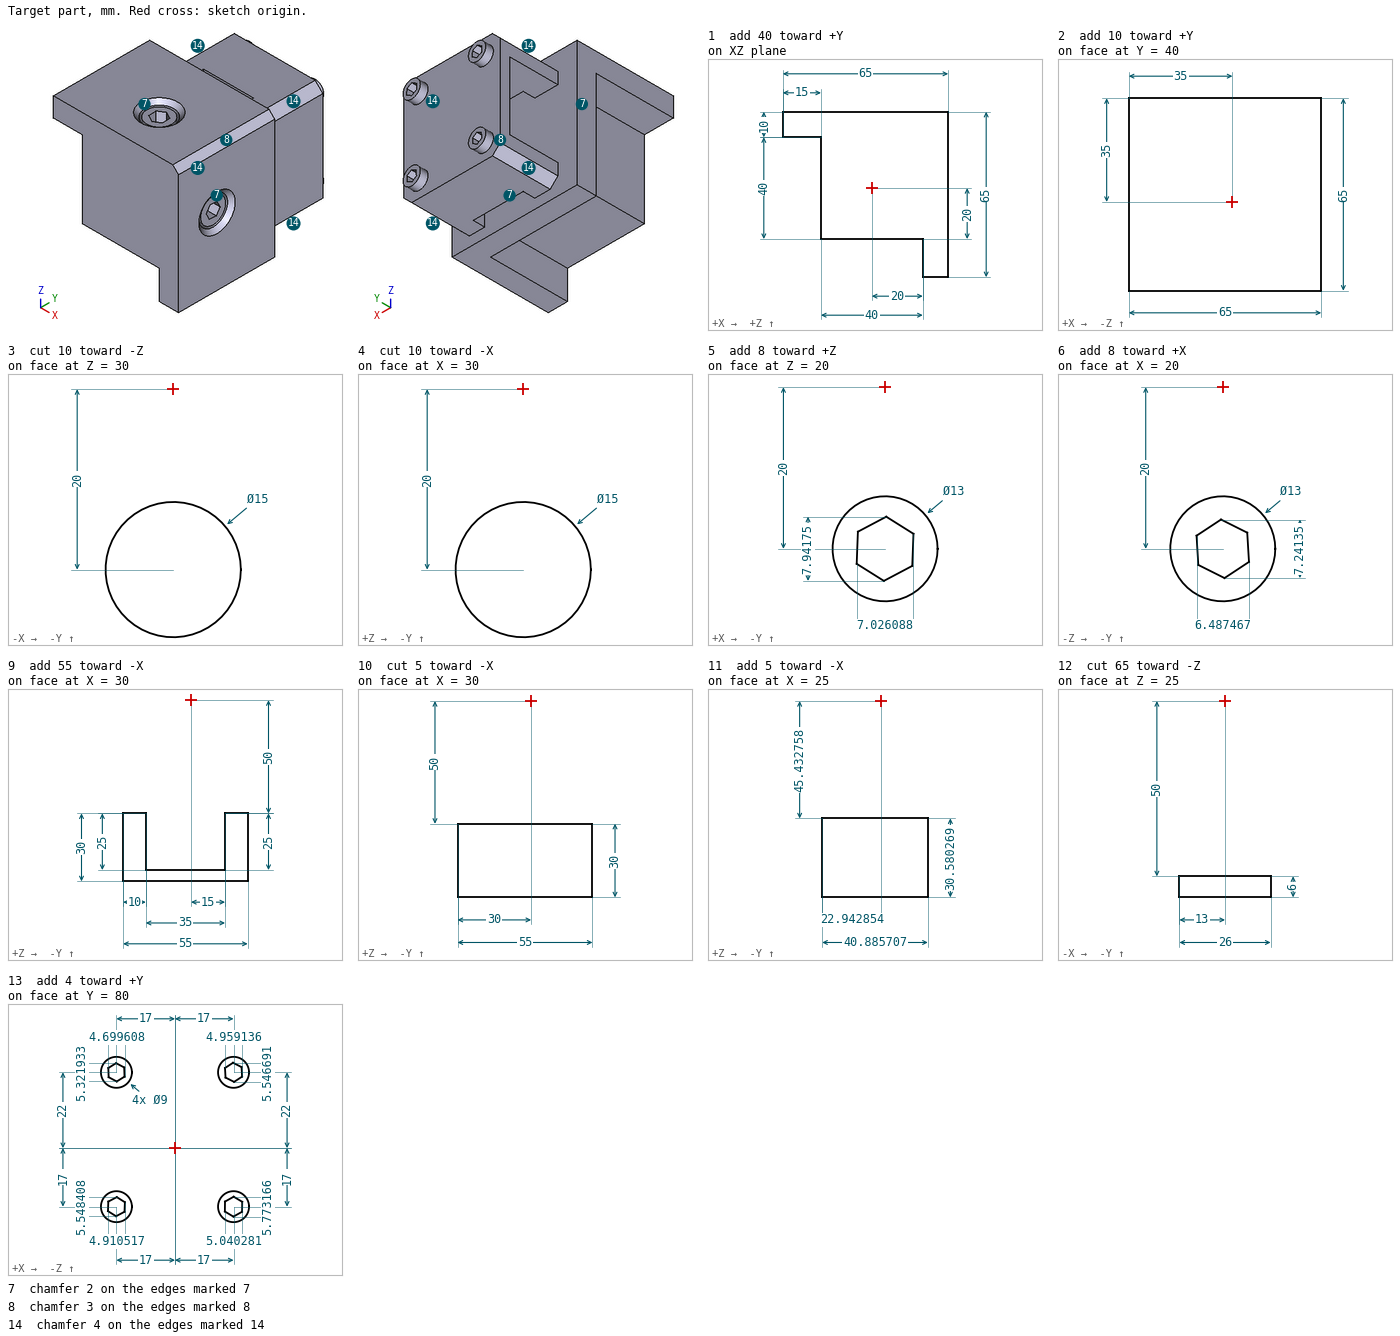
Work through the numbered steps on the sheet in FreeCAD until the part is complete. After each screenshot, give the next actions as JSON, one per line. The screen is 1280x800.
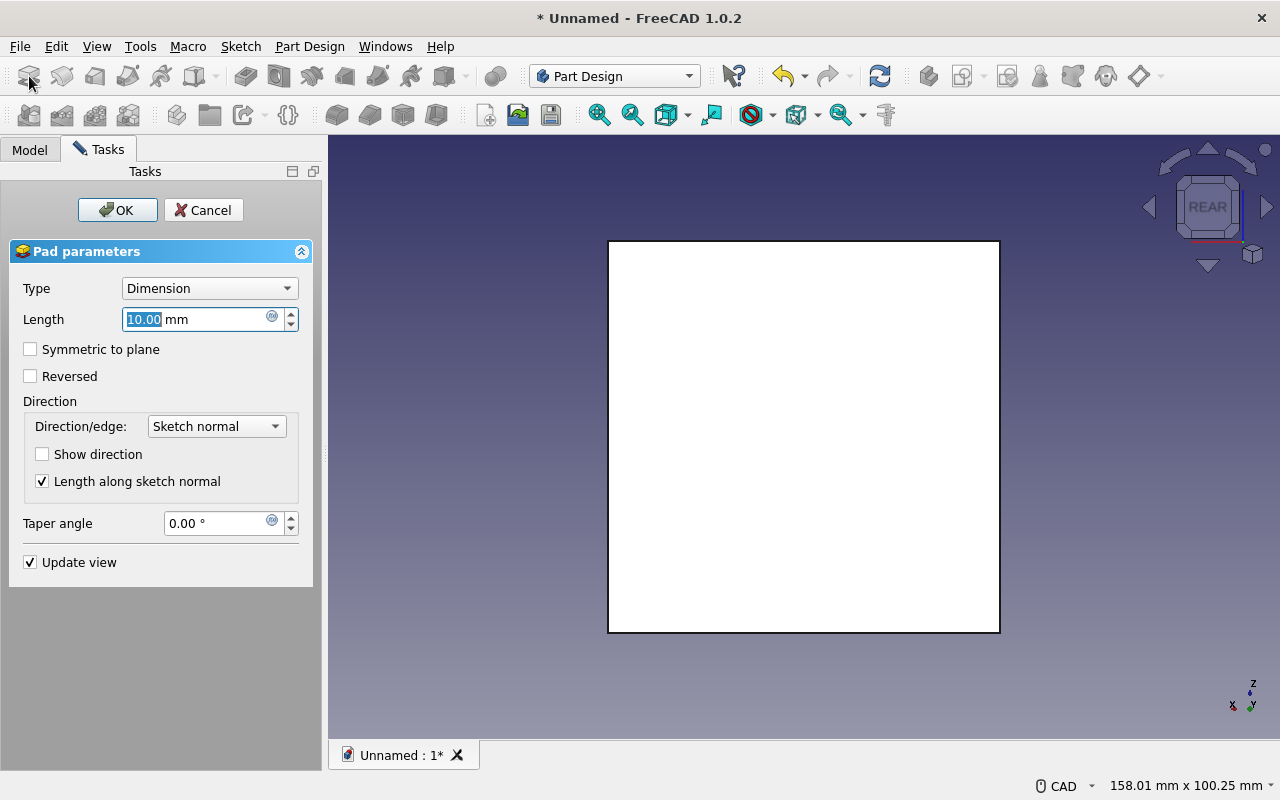
{"action": "type", "text": "10"}
{"action": "key", "text": "Tab"}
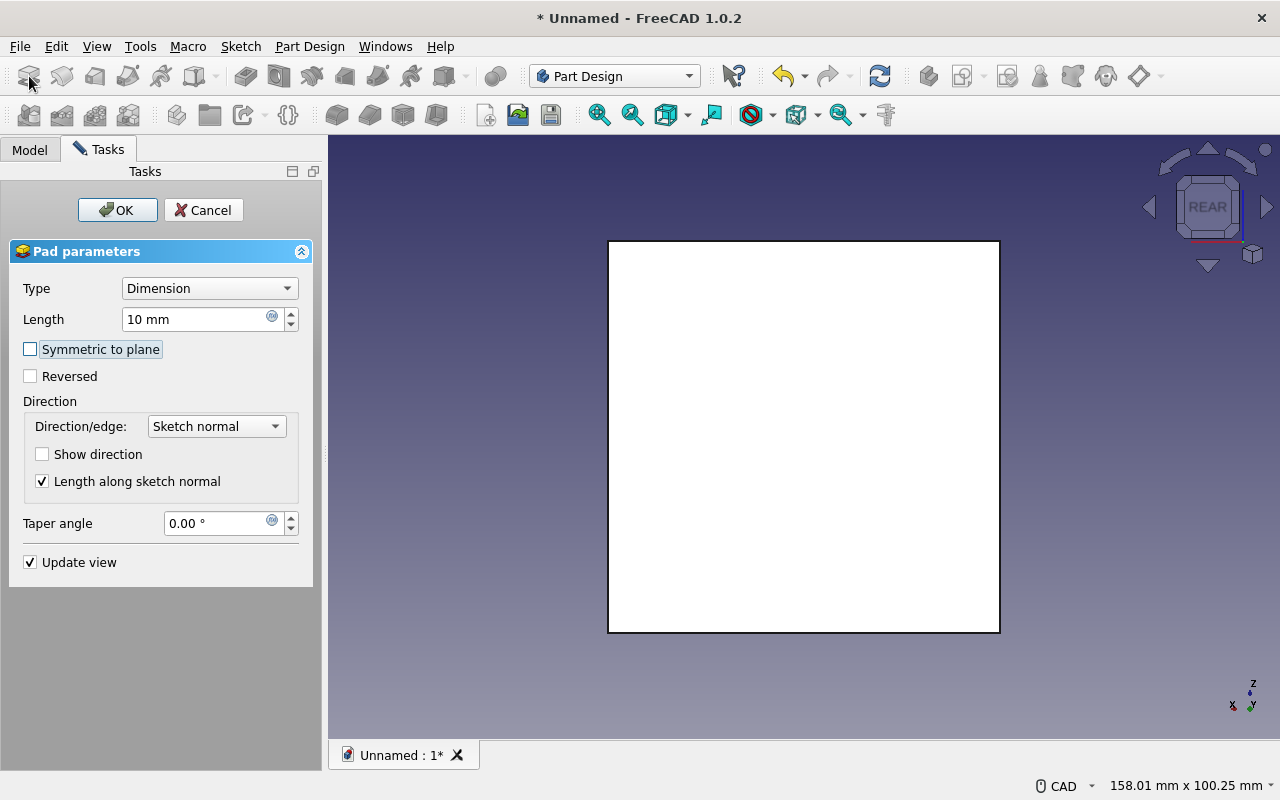
{"action": "left_click", "coordinate": [118, 210]}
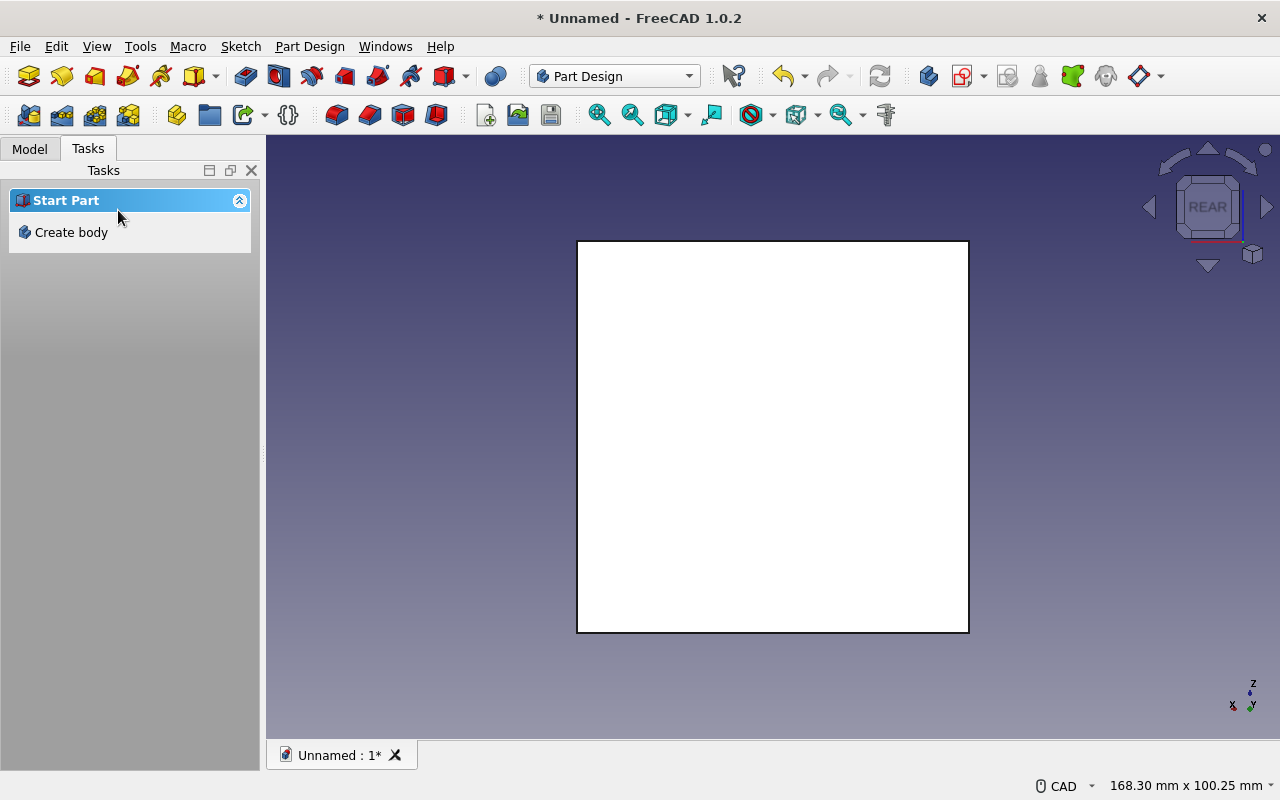
{"action": "key", "text": "0"}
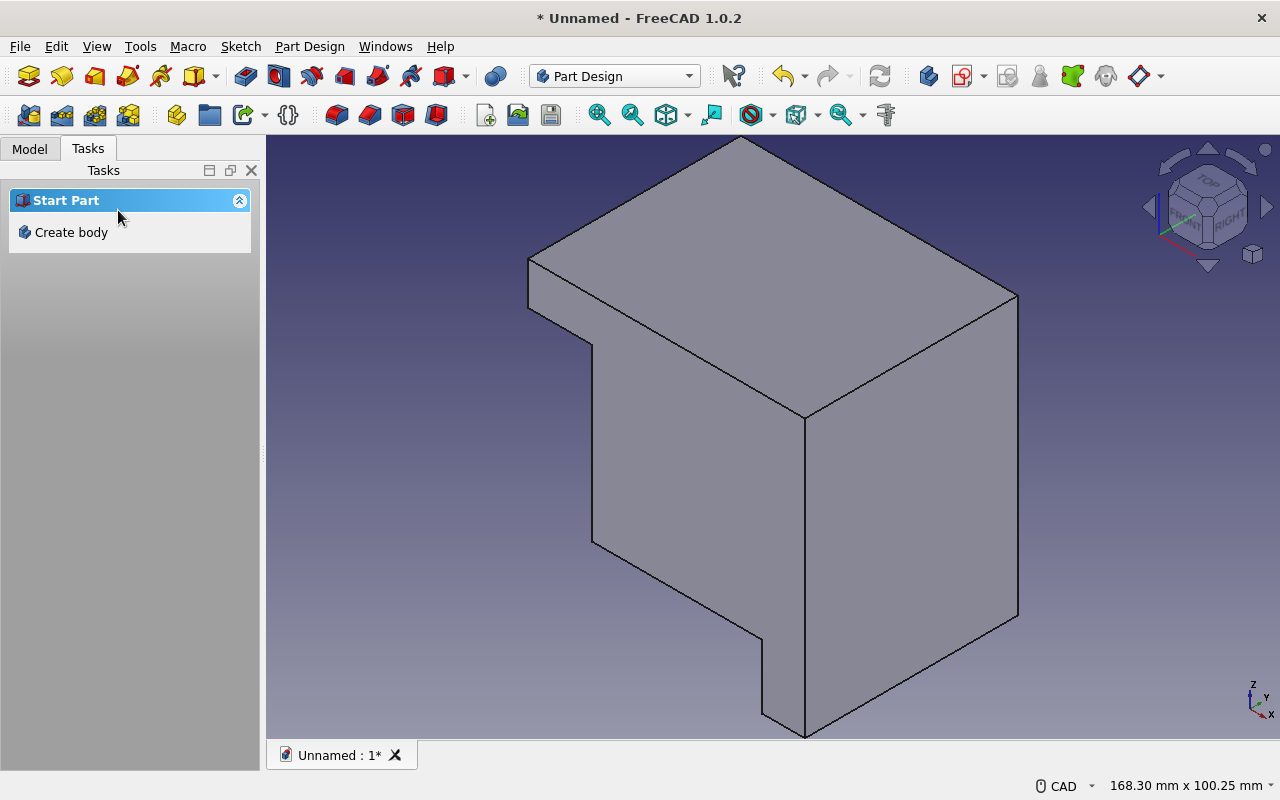
{"action": "left_click", "coordinate": [773, 276]}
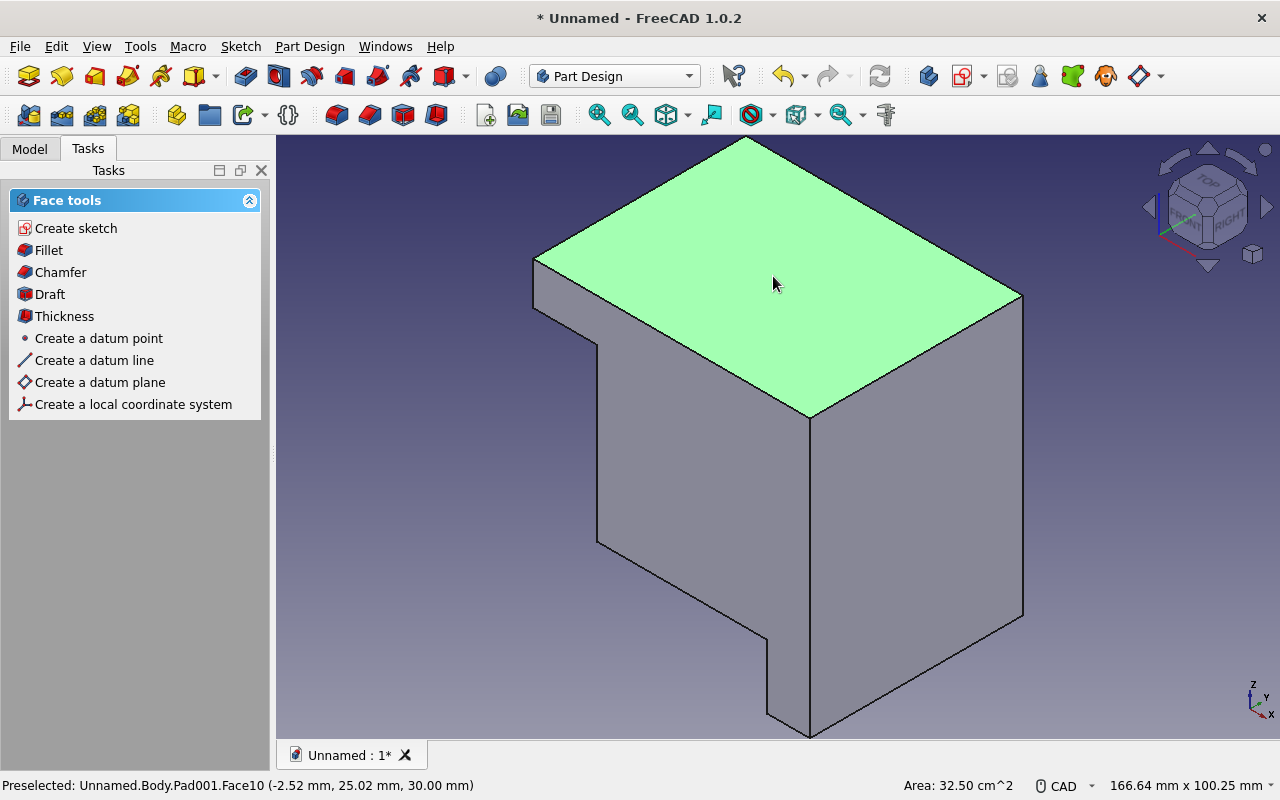
{"action": "left_click", "coordinate": [962, 76]}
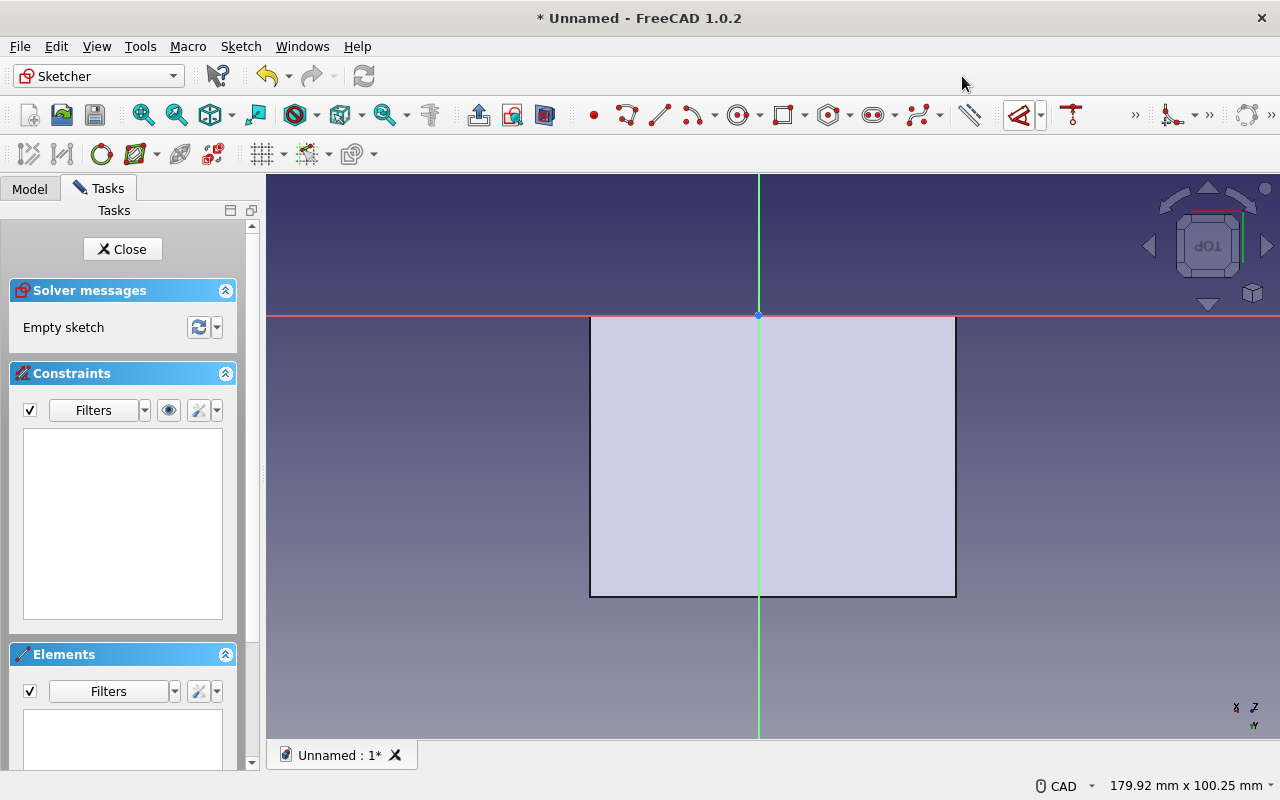
{"action": "scroll", "coordinate": [803, 341], "scroll_direction": "up", "scroll_amount": 4}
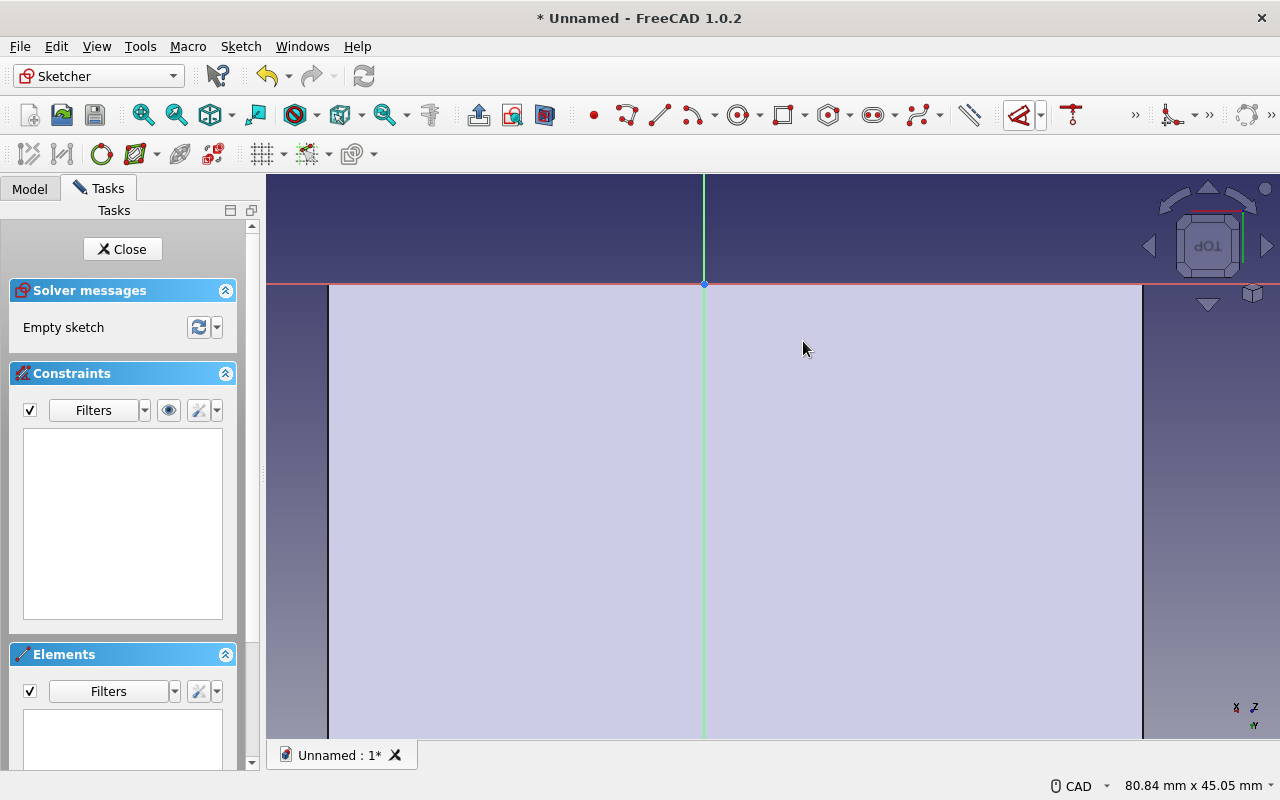
{"action": "left_click", "coordinate": [738, 116]}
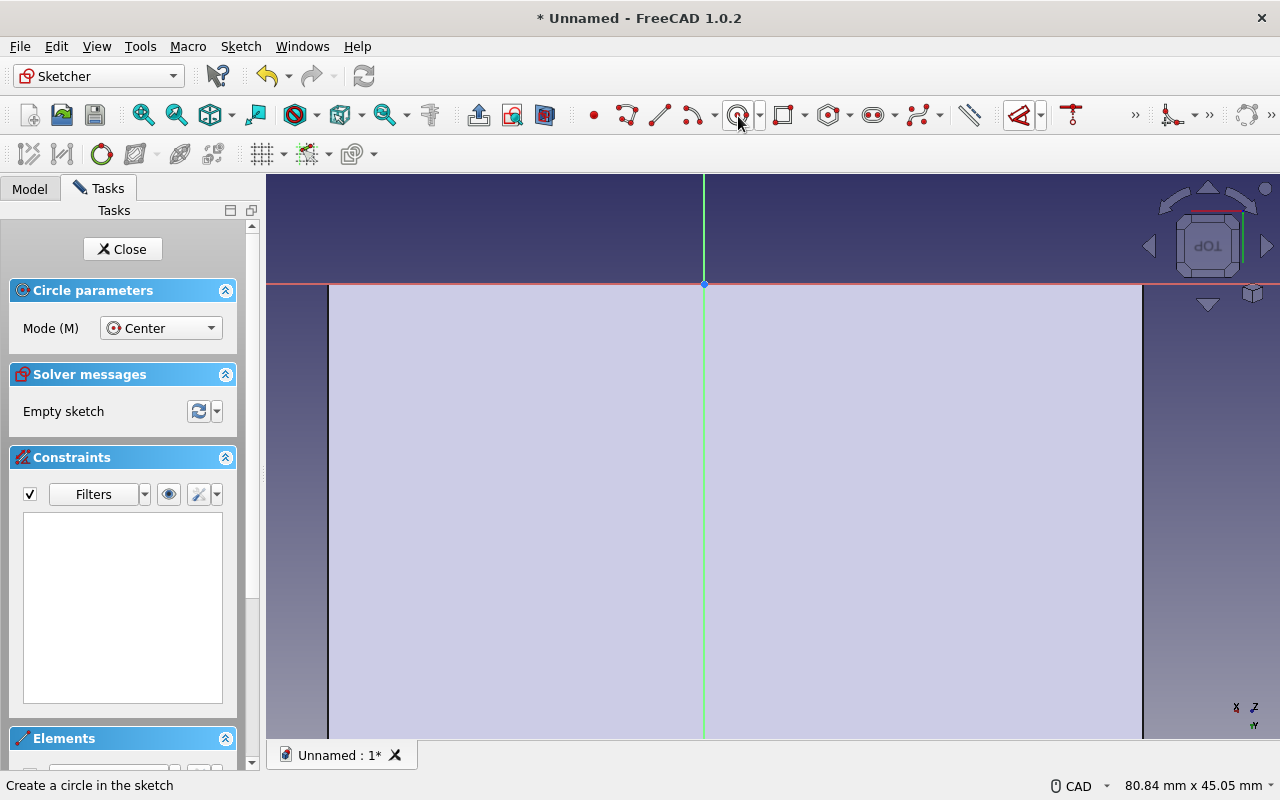
{"action": "left_click", "coordinate": [704, 535]}
{"action": "mouse_move", "coordinate": [771, 468]}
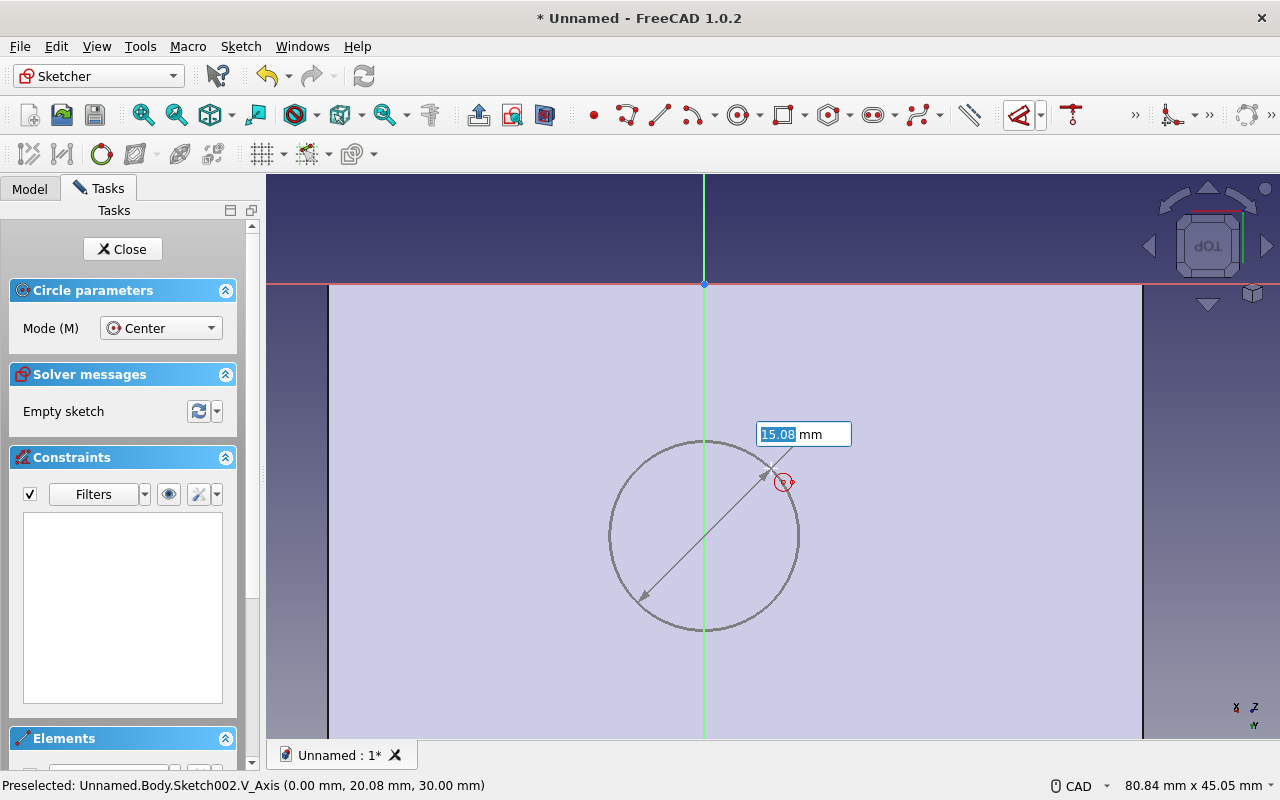
{"action": "type", "text": "15"}
{"action": "key", "text": "Return"}
{"action": "key", "text": "Escape"}